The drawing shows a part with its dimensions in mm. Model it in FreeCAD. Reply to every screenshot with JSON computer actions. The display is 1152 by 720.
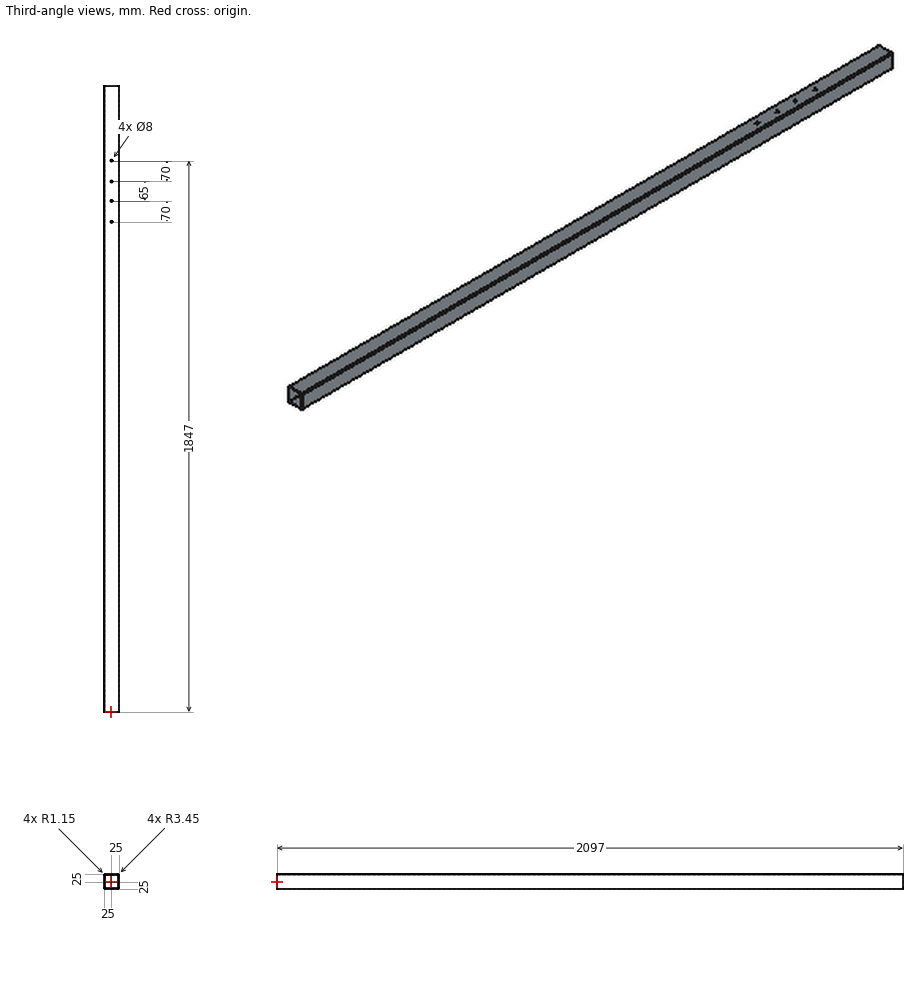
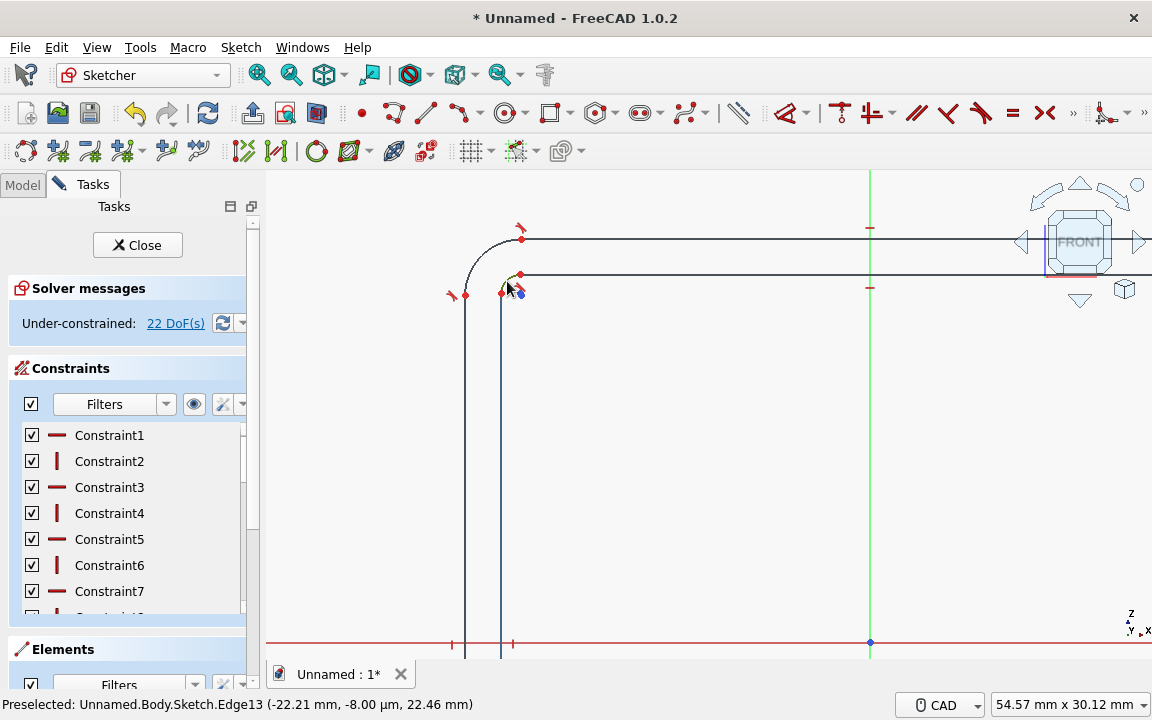
{"action": "left_click", "coordinate": [982, 114]}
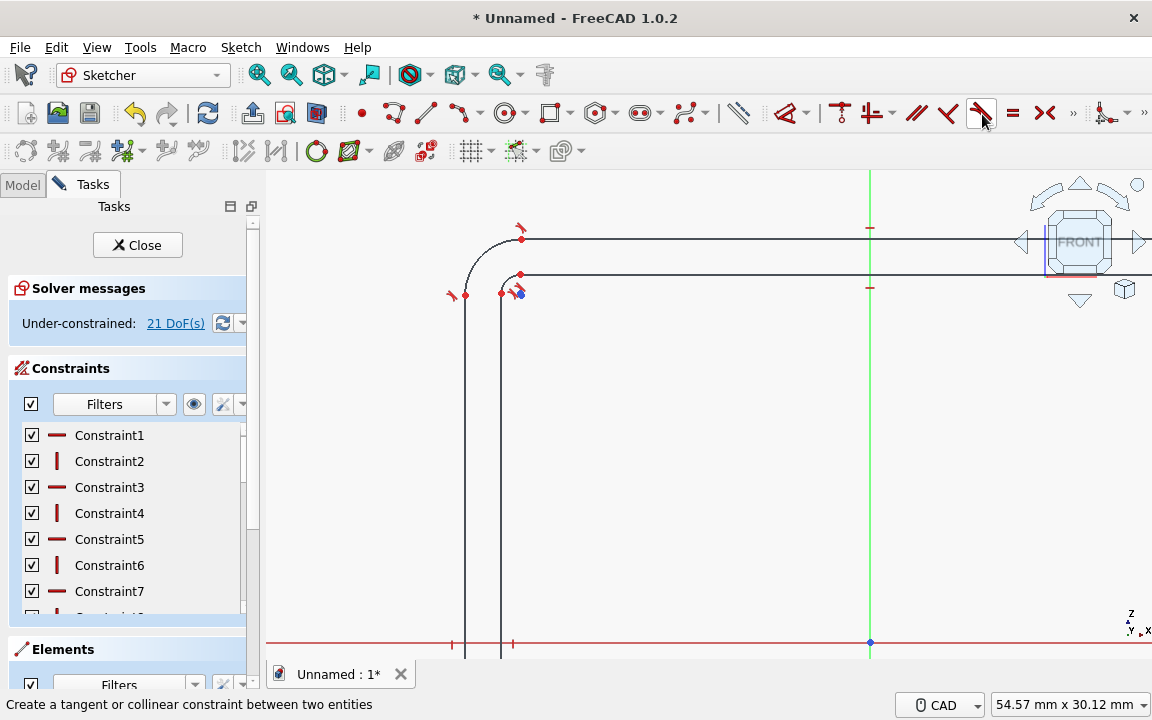
{"action": "left_click", "coordinate": [501, 504]}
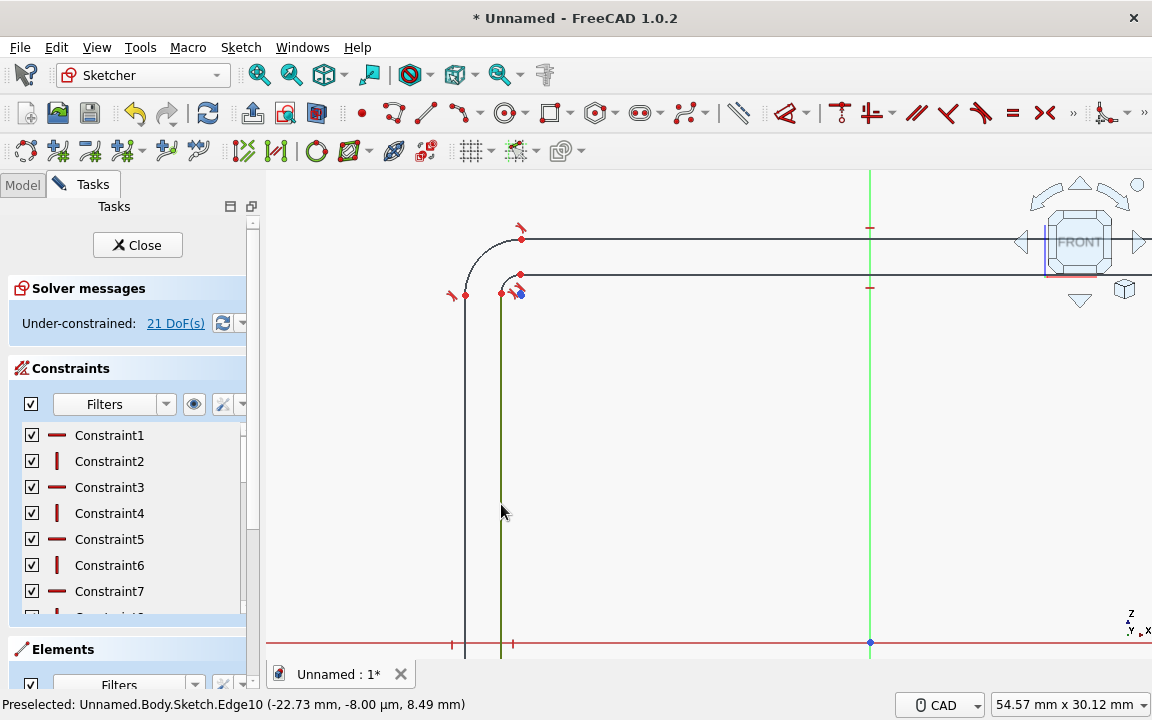
{"action": "scroll", "coordinate": [507, 282], "scroll_direction": "down", "scroll_amount": 5}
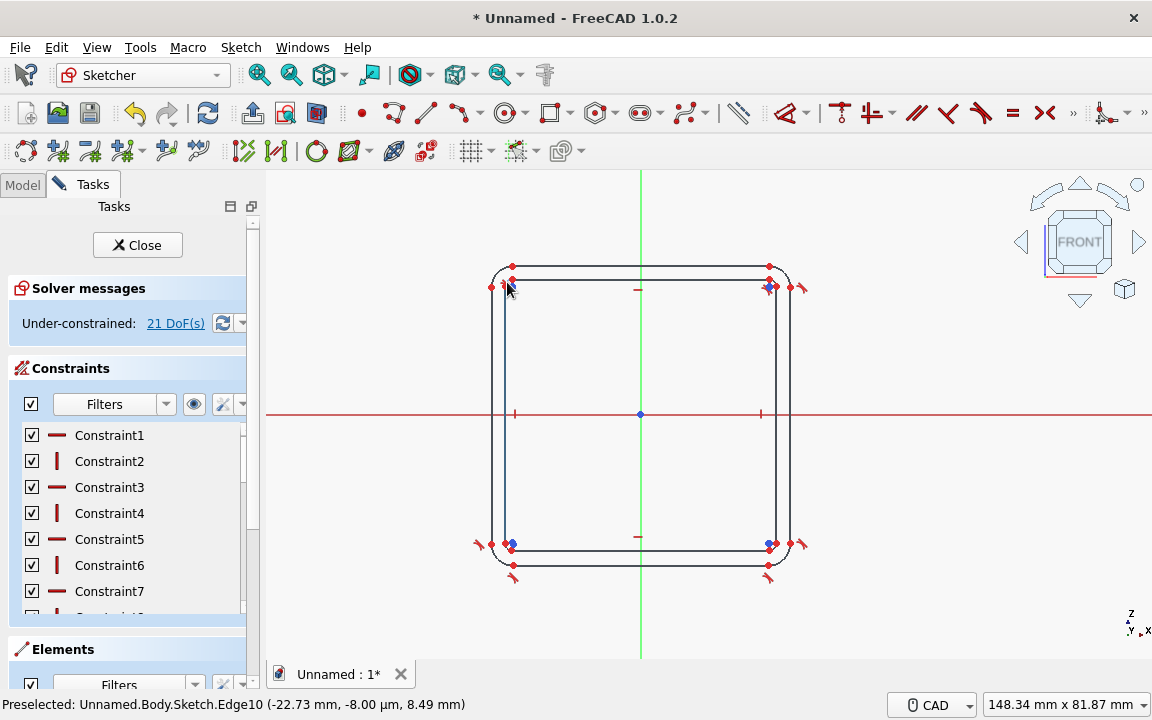
{"action": "scroll", "coordinate": [507, 549], "scroll_direction": "up", "scroll_amount": 5}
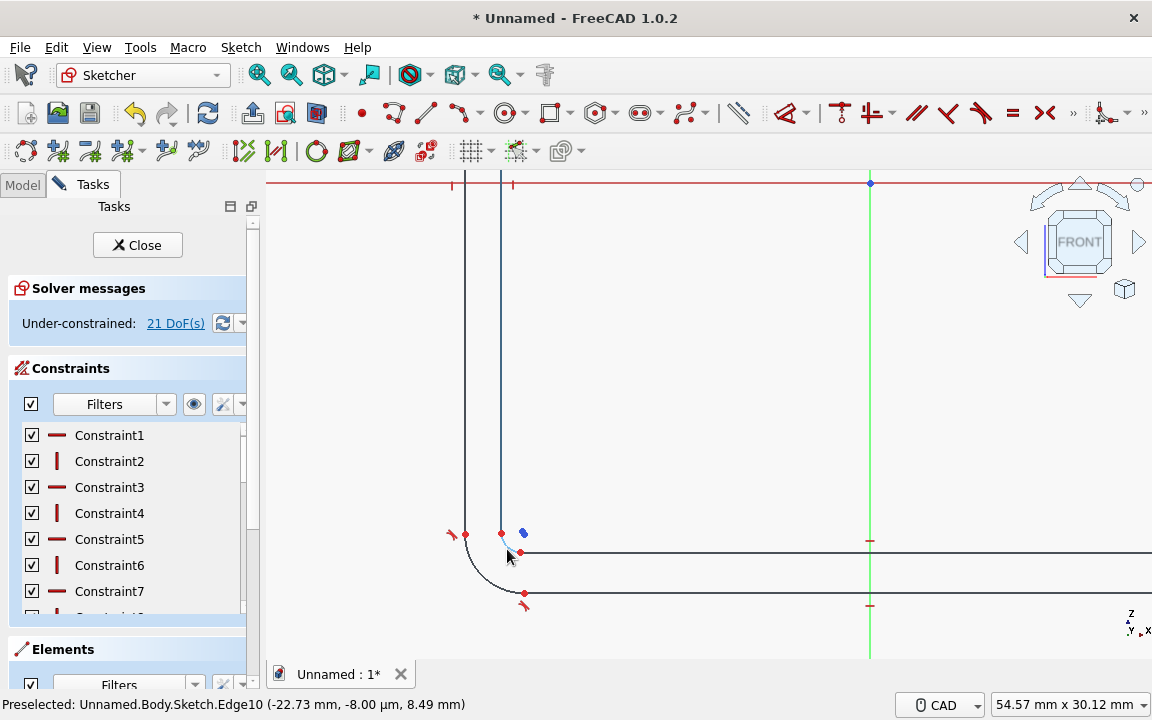
{"action": "left_click", "coordinate": [507, 547]}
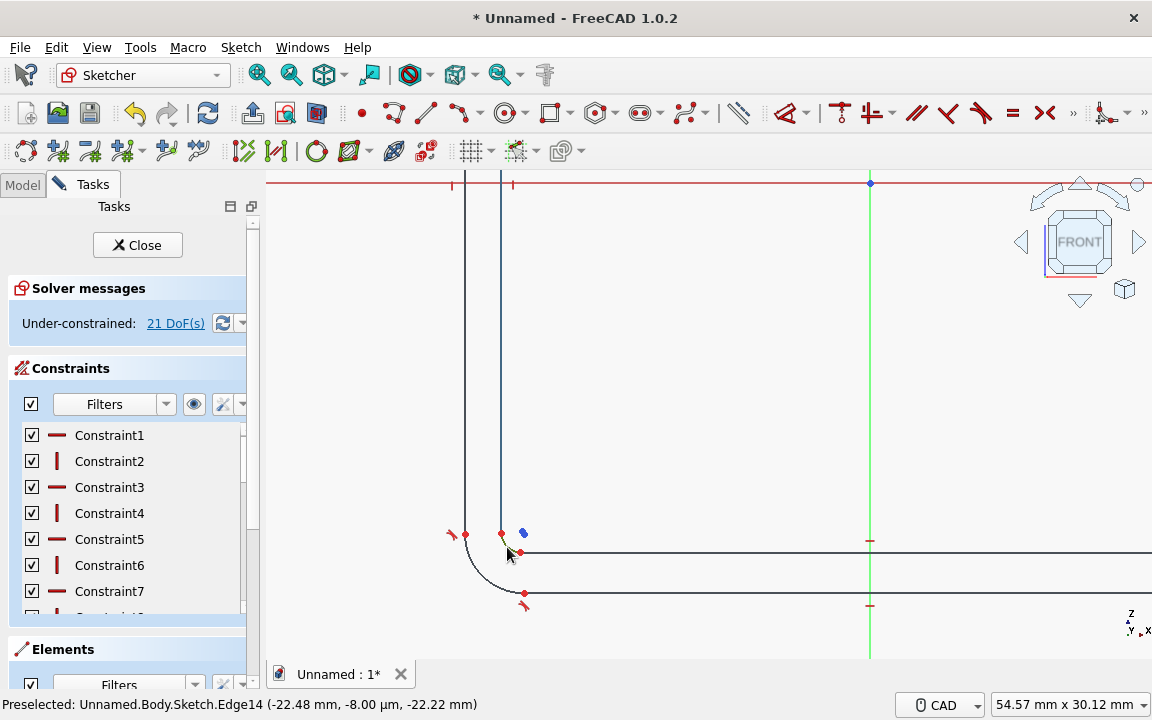
{"action": "left_click", "coordinate": [982, 114]}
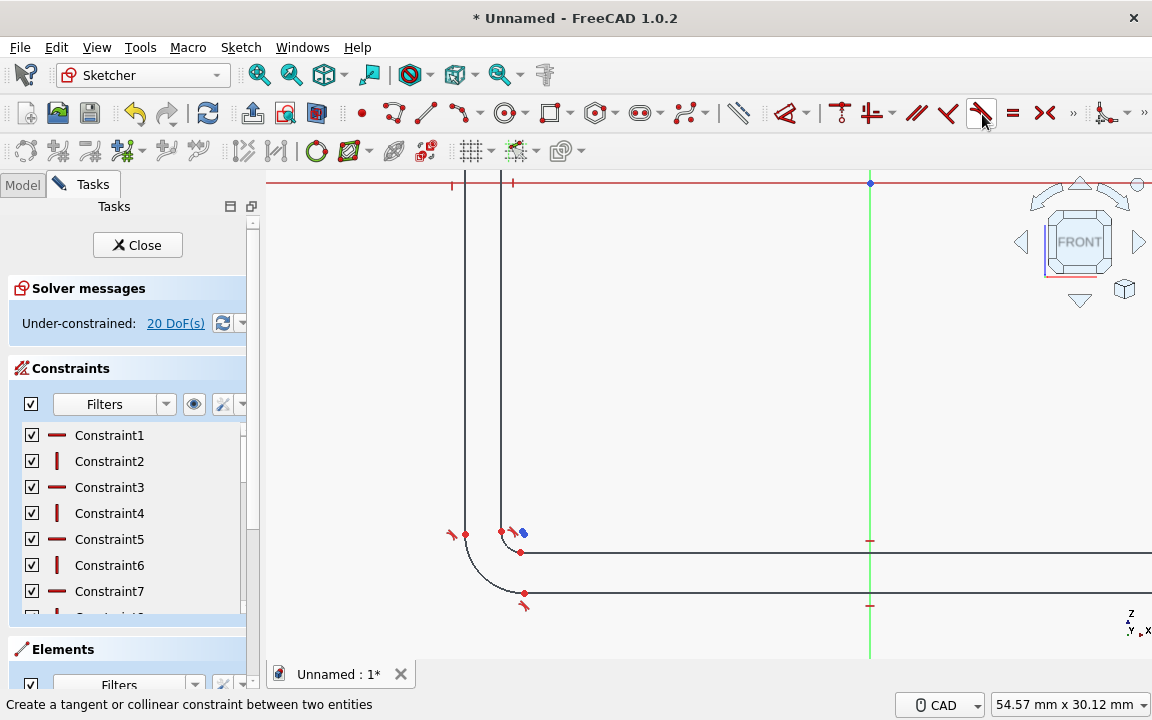
{"action": "left_click", "coordinate": [730, 553]}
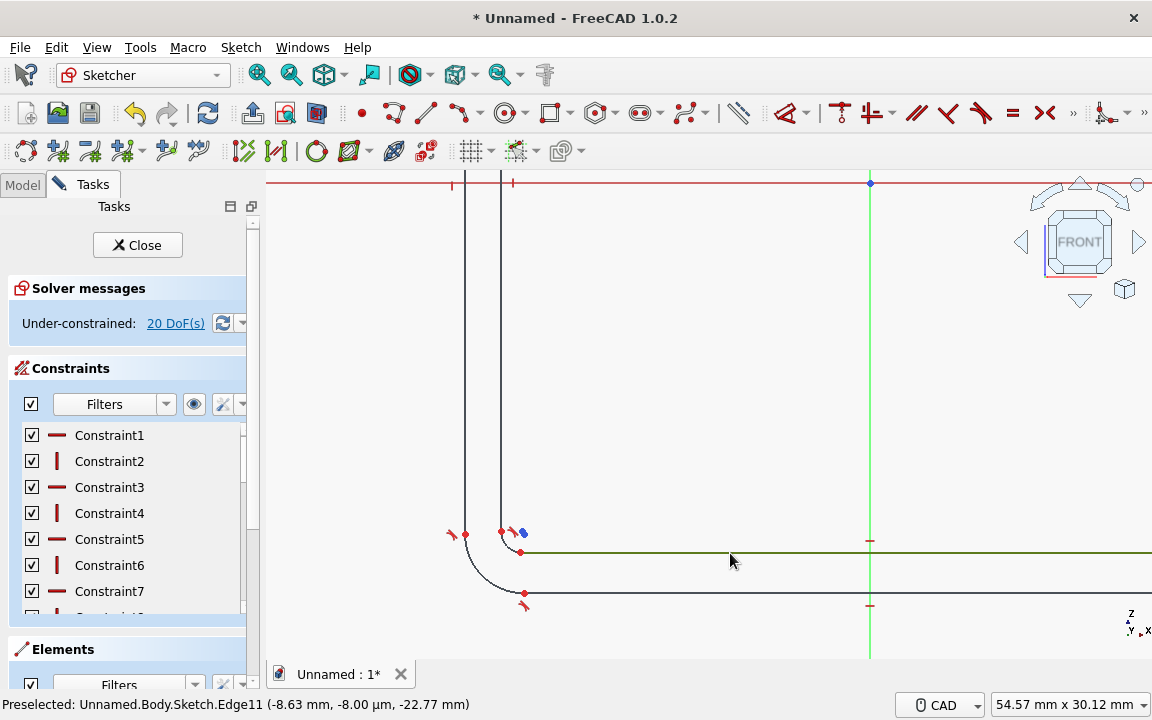
{"action": "scroll", "coordinate": [503, 541], "scroll_direction": "up", "scroll_amount": 2}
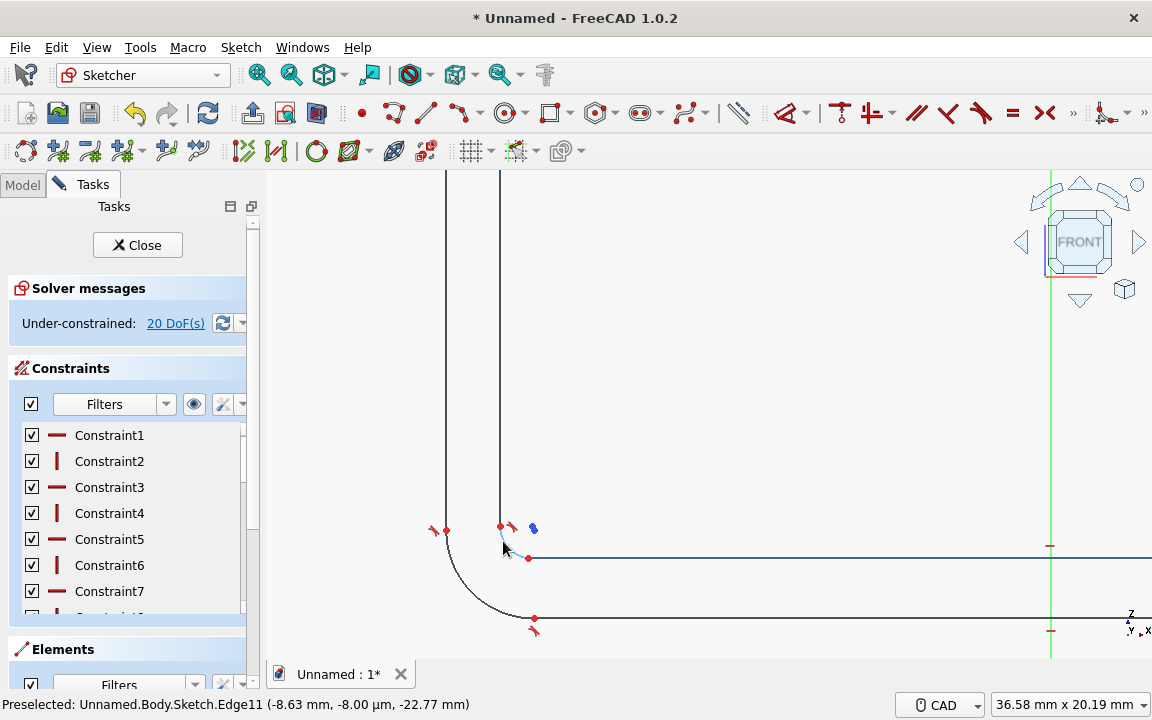
{"action": "left_click", "coordinate": [503, 540]}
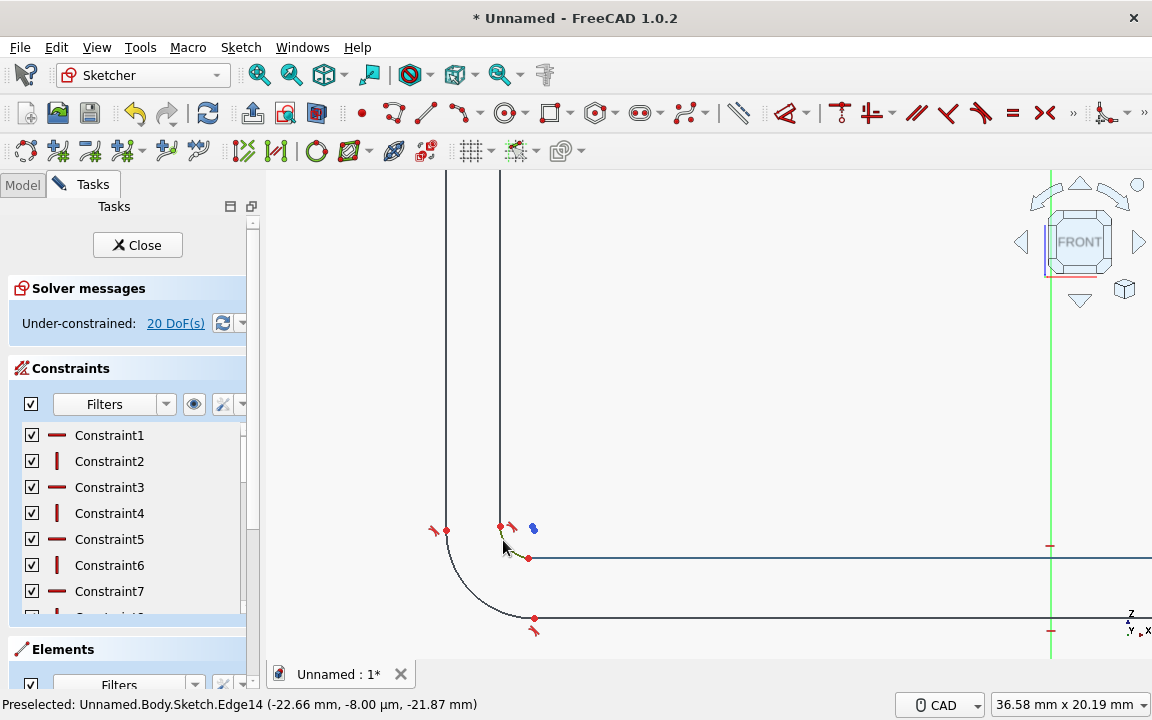
{"action": "left_click", "coordinate": [982, 114]}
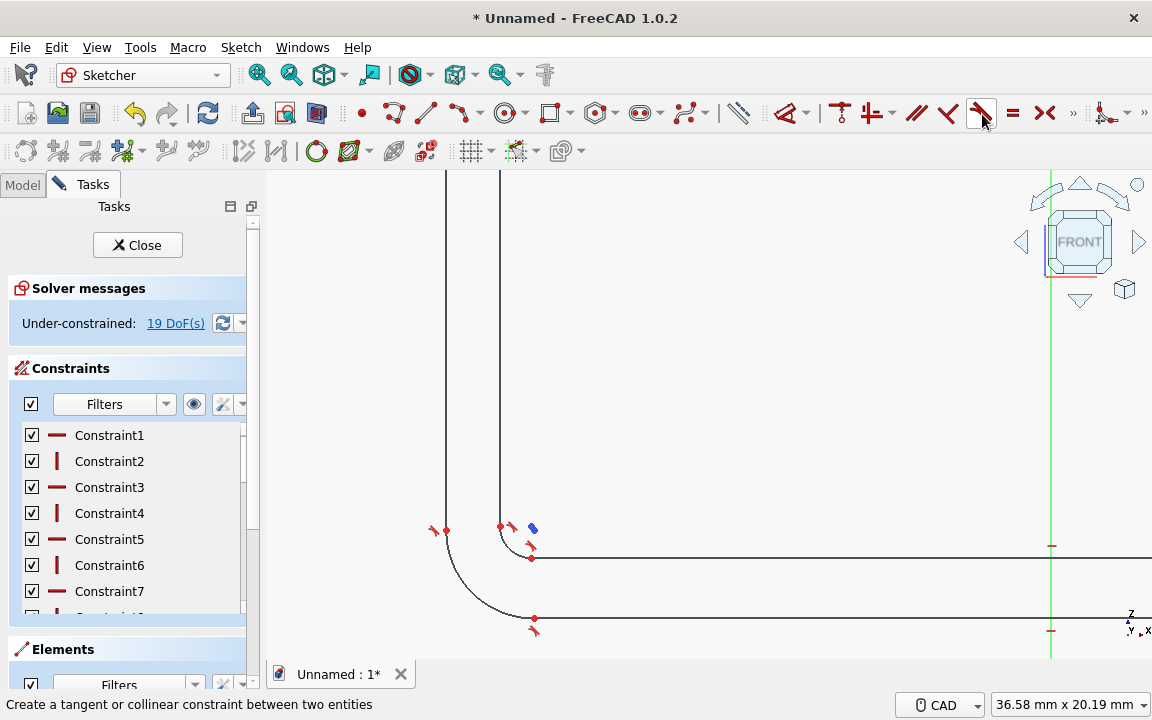
{"action": "scroll", "coordinate": [506, 548], "scroll_direction": "down", "scroll_amount": 7}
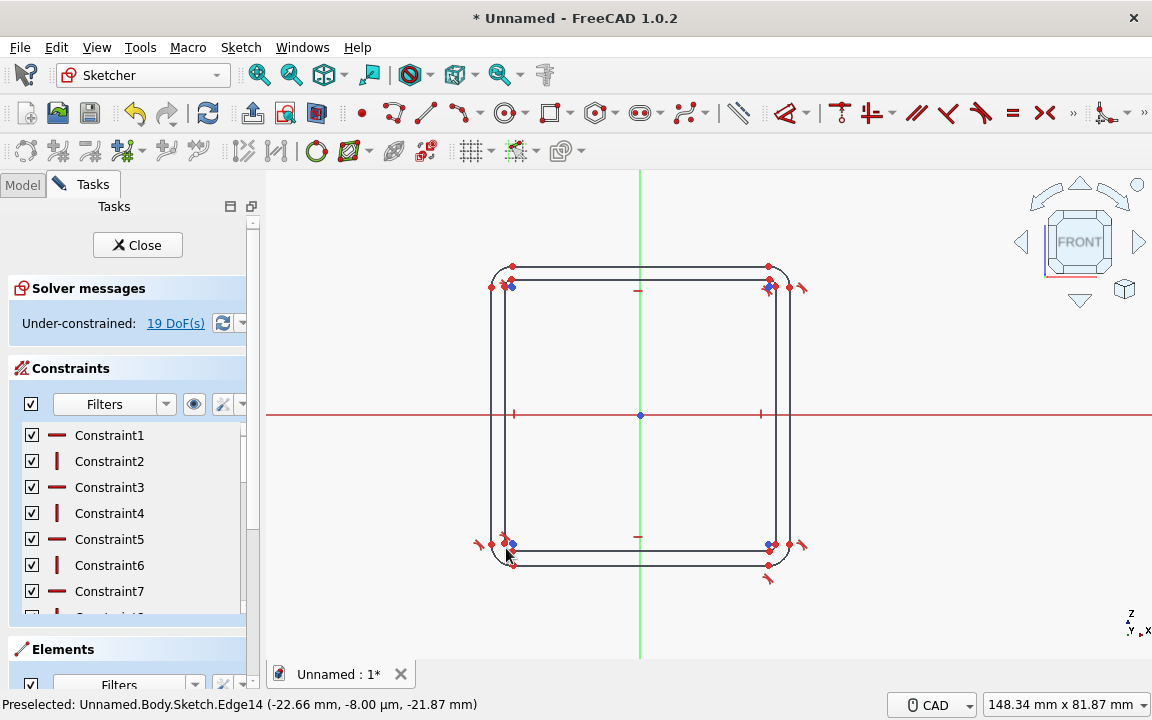
{"action": "left_click", "coordinate": [590, 551]}